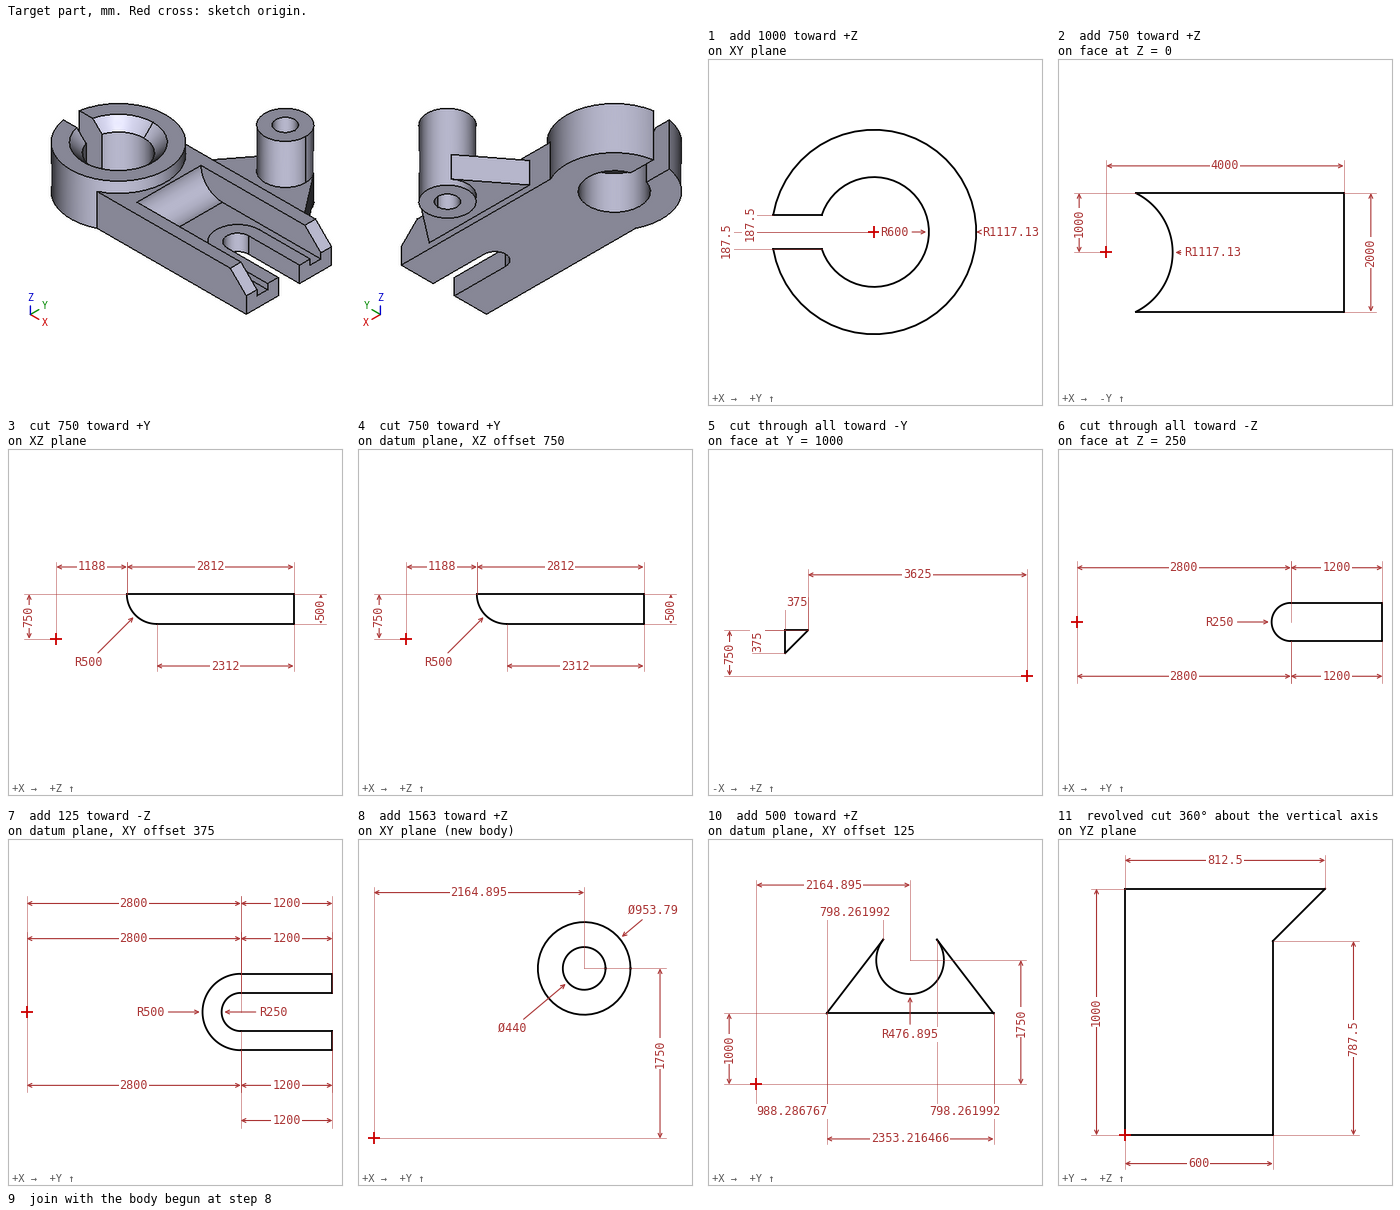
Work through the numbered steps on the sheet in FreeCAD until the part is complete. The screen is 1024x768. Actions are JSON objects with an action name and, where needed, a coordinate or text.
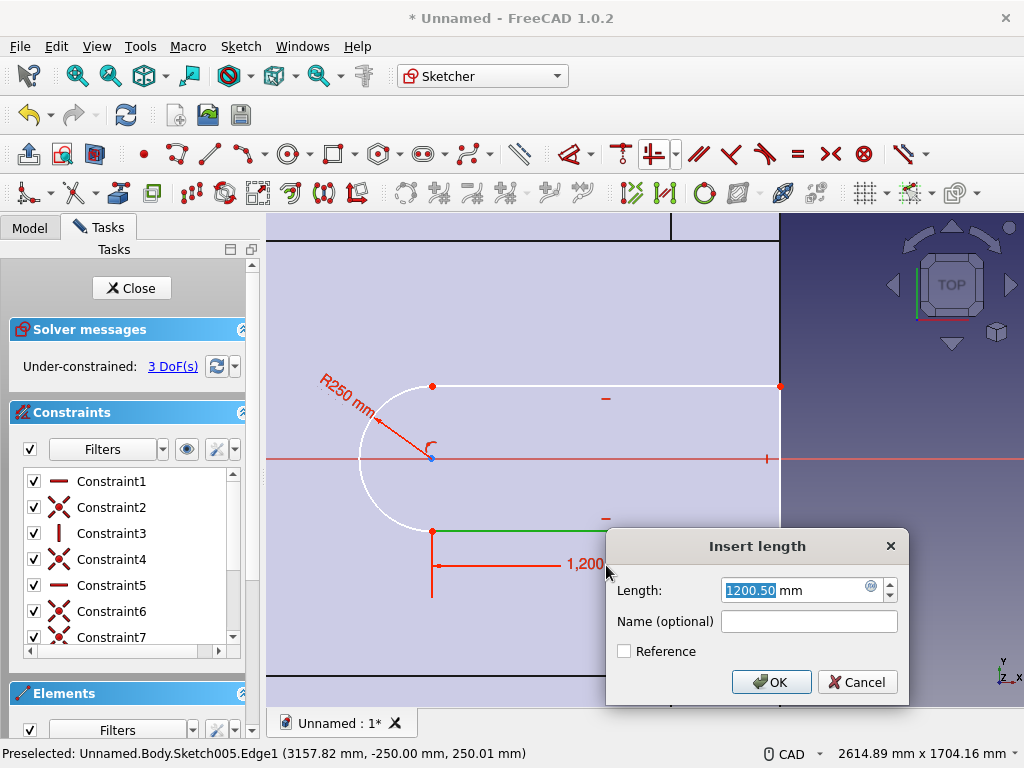
{"action": "type", "text": "1200"}
{"action": "key", "text": "Return"}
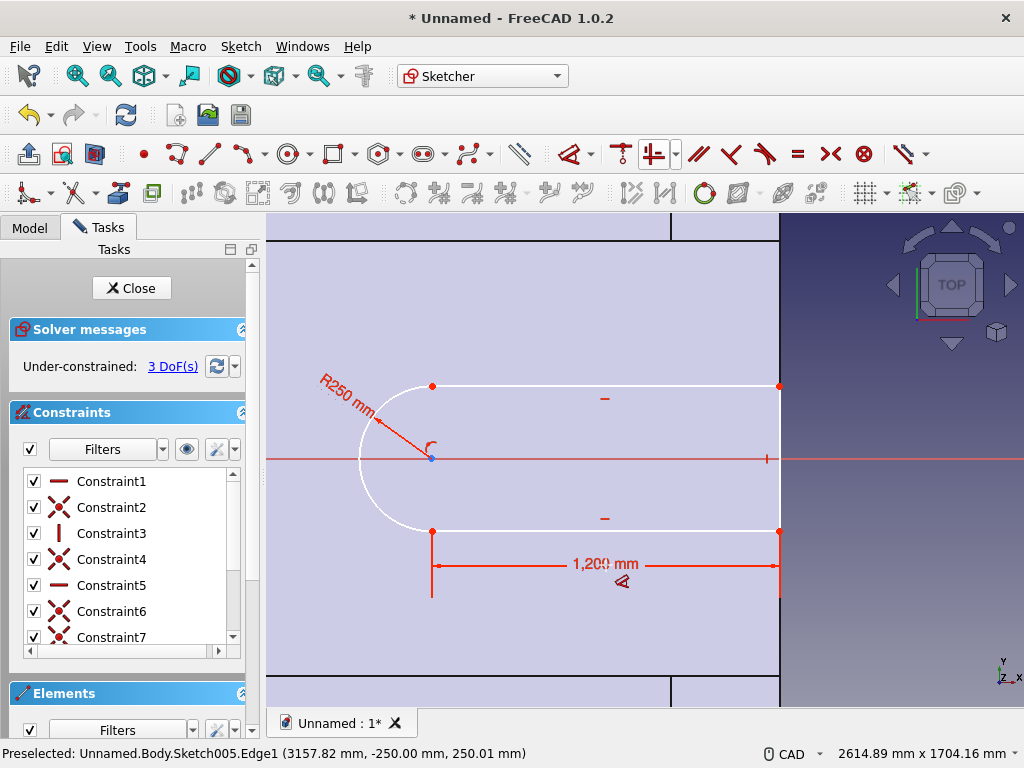
{"action": "left_click", "coordinate": [676, 386]}
{"action": "left_click", "coordinate": [606, 352]}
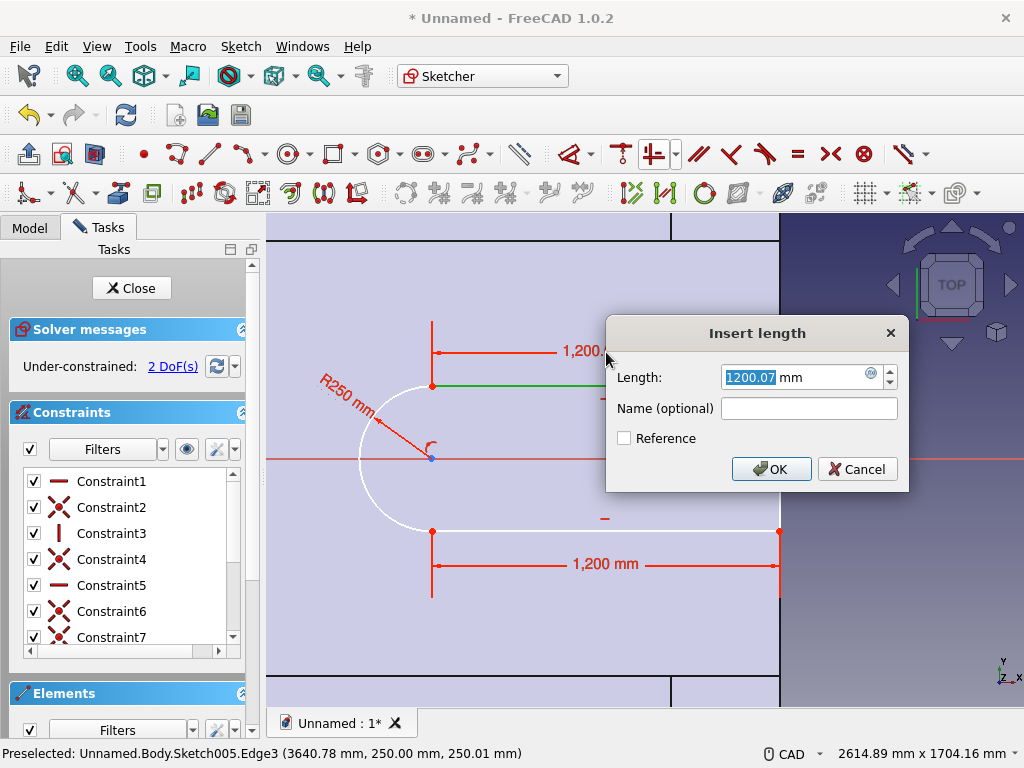
{"action": "type", "text": "1200"}
{"action": "key", "text": "Return"}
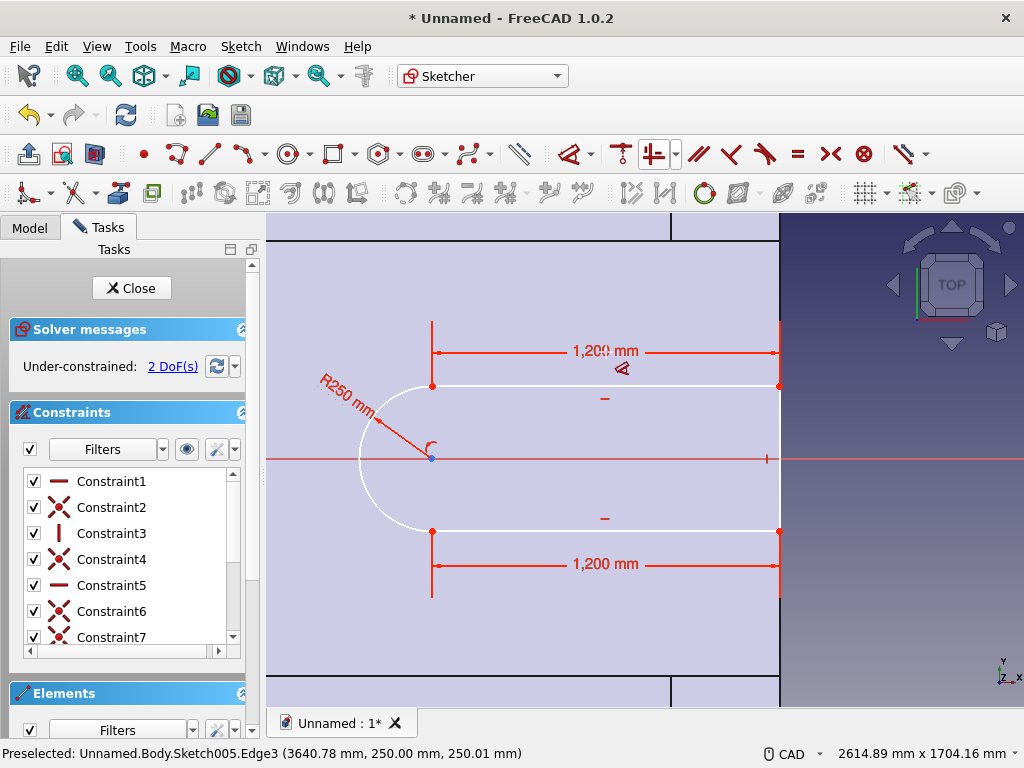
{"action": "left_click", "coordinate": [432, 531]}
{"action": "left_click", "coordinate": [363, 565]}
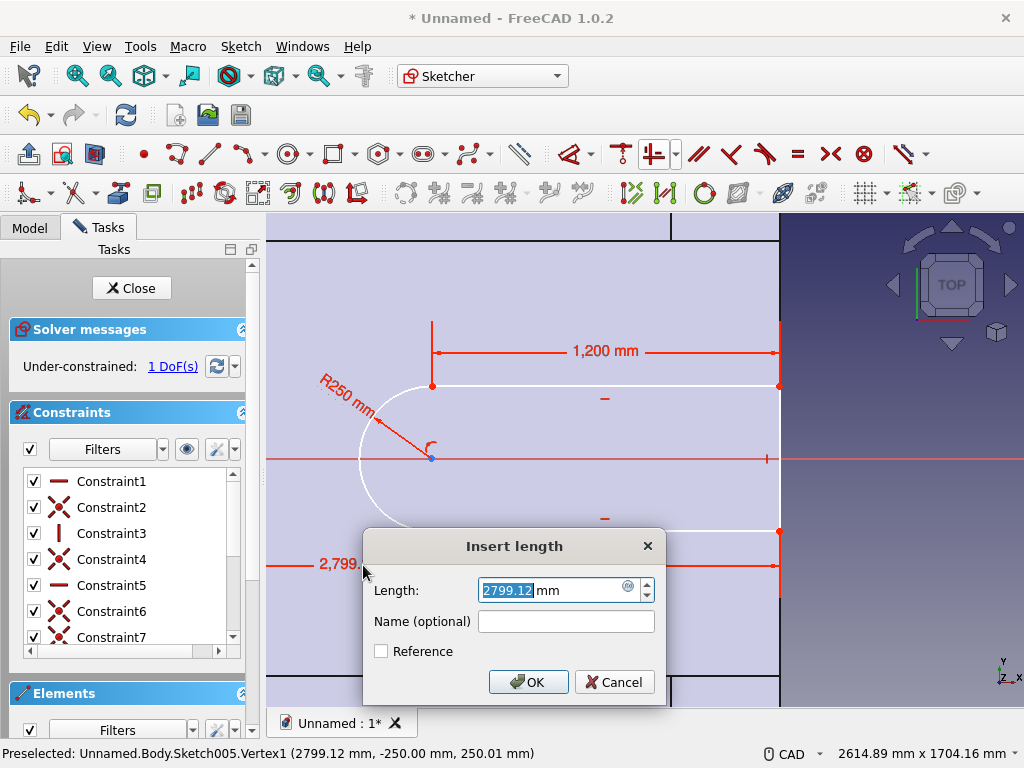
{"action": "type", "text": "2800"}
{"action": "key", "text": "Return"}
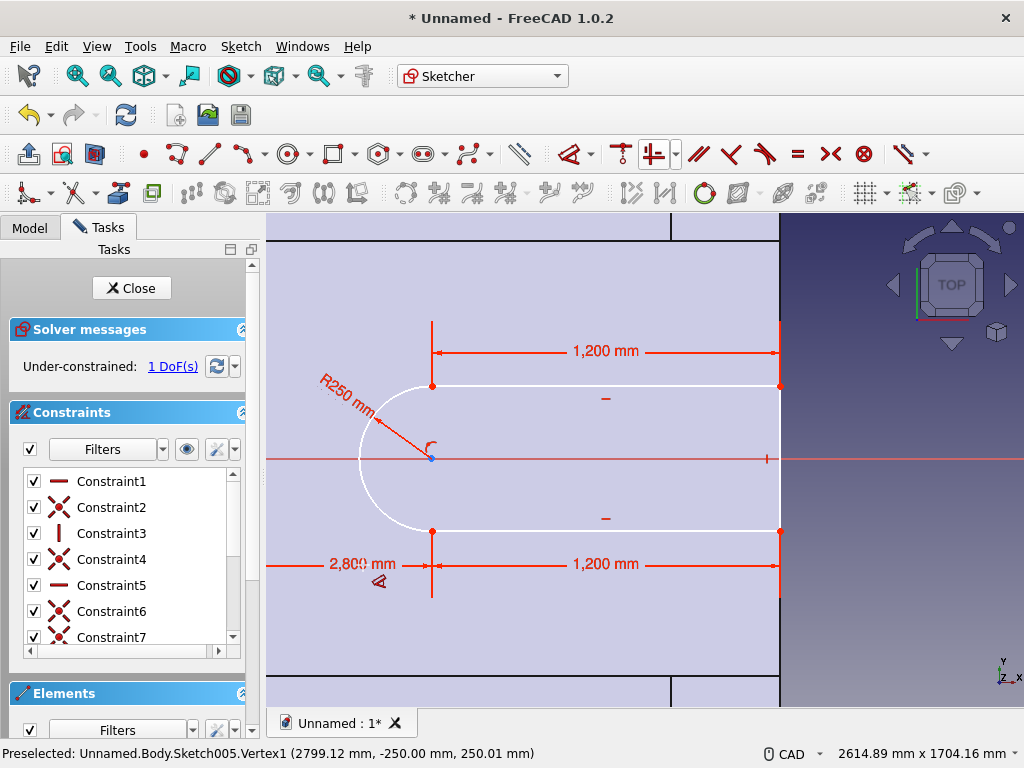
{"action": "left_click", "coordinate": [432, 459]}
{"action": "left_click", "coordinate": [331, 493]}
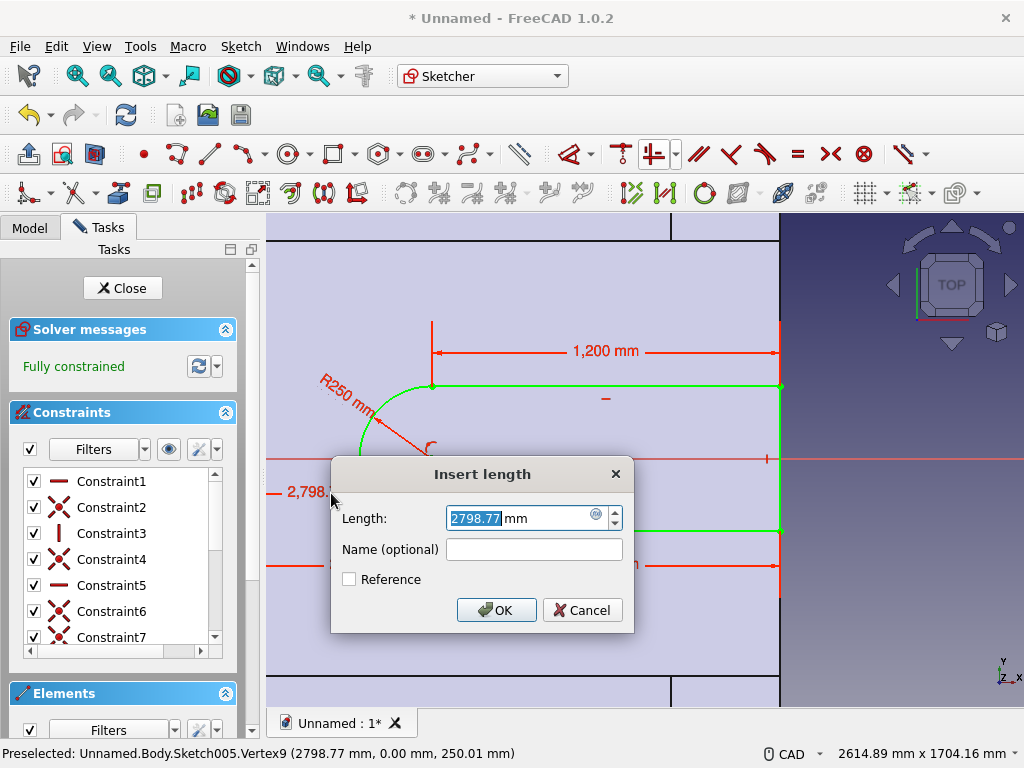
{"action": "type", "text": "2800"}
{"action": "key", "text": "Return"}
{"action": "key", "text": "Escape"}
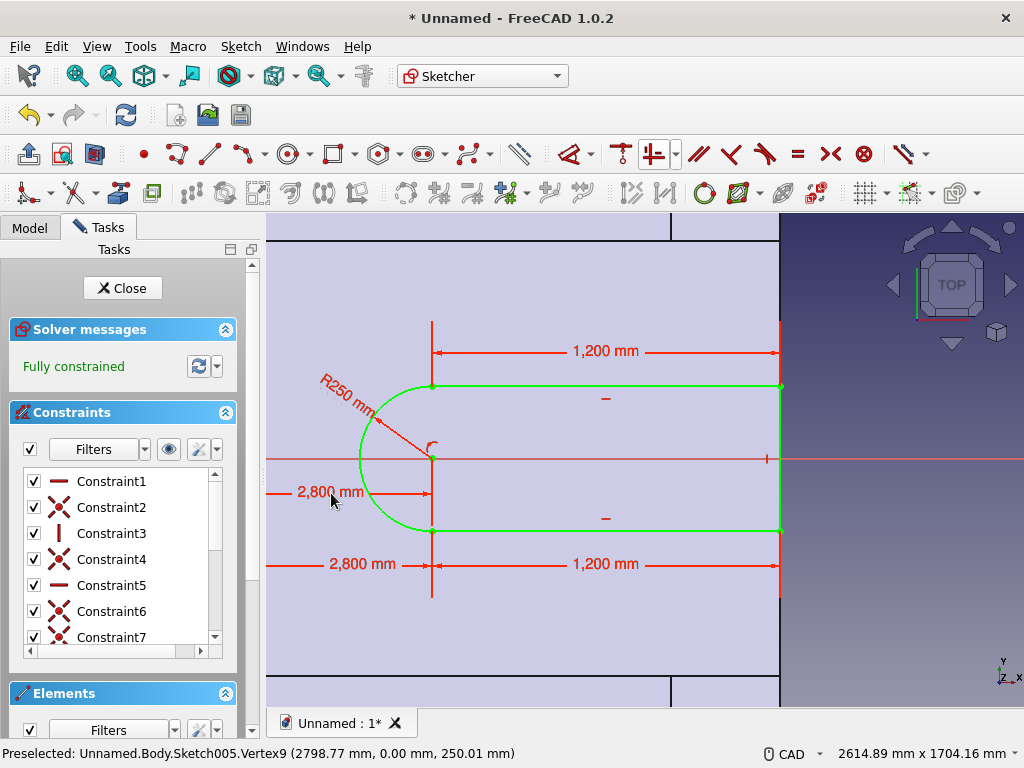
{"action": "left_click", "coordinate": [123, 288]}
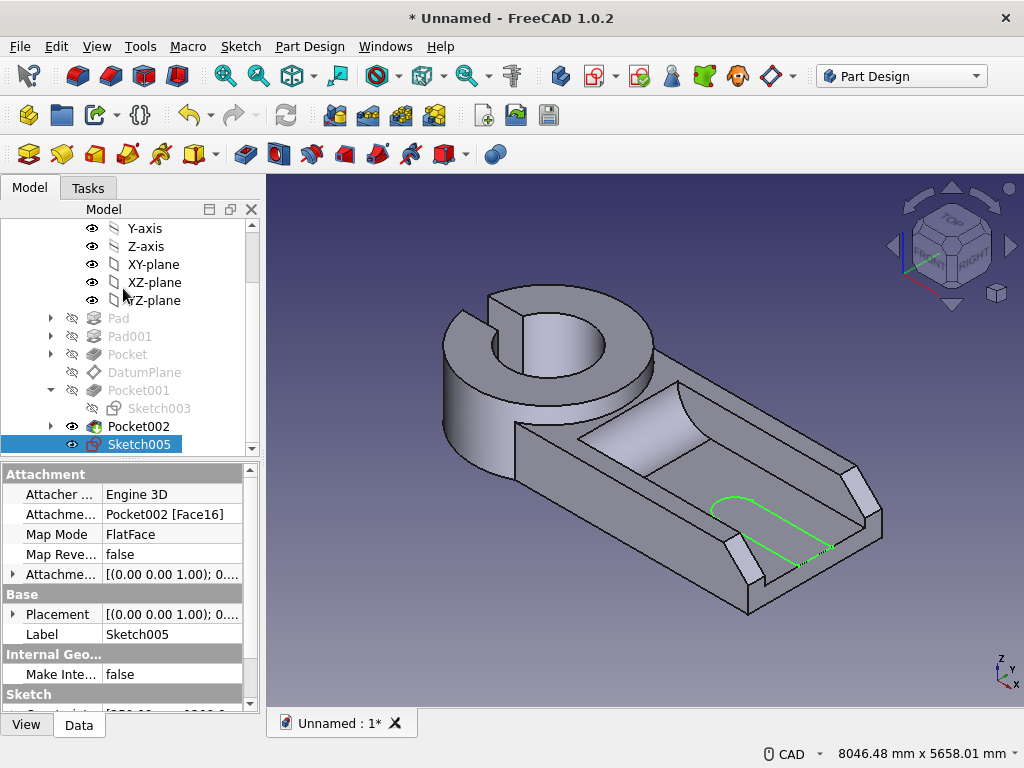
{"action": "left_click", "coordinate": [246, 154]}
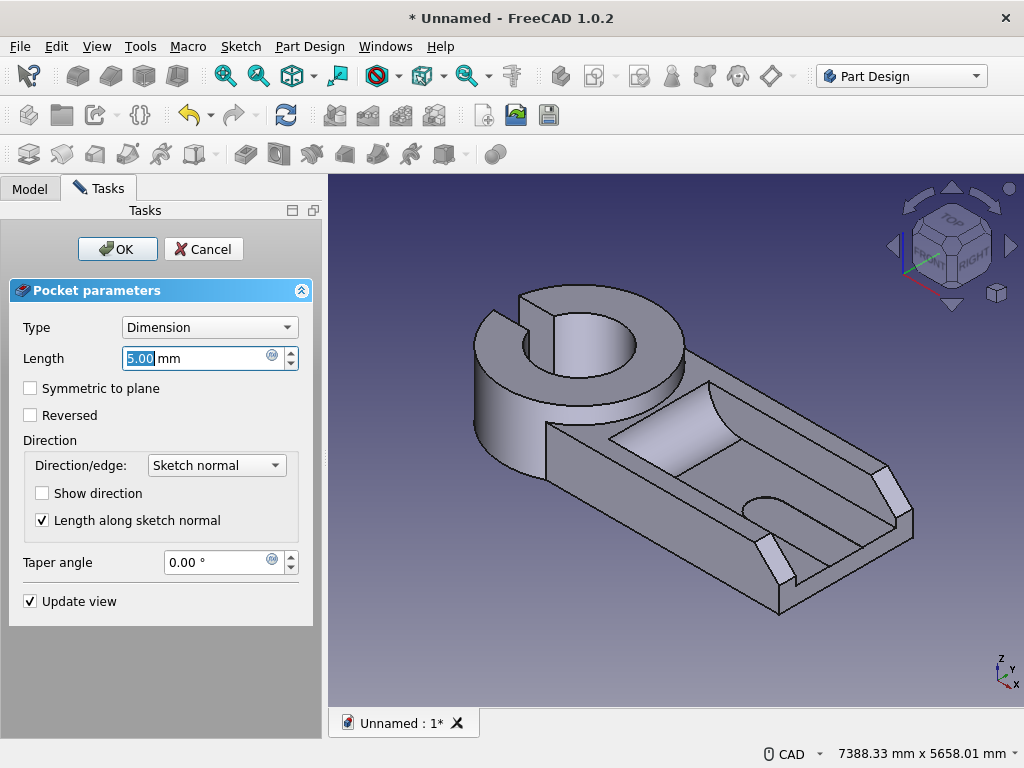
{"action": "left_click", "coordinate": [210, 328]}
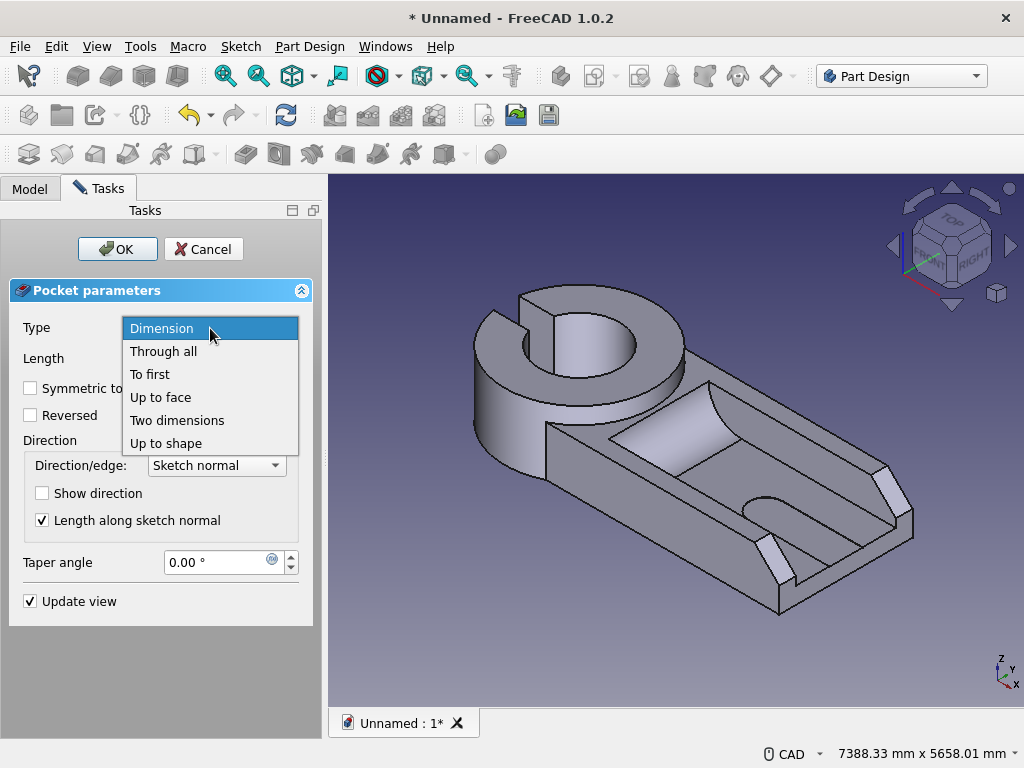
{"action": "left_click", "coordinate": [208, 352]}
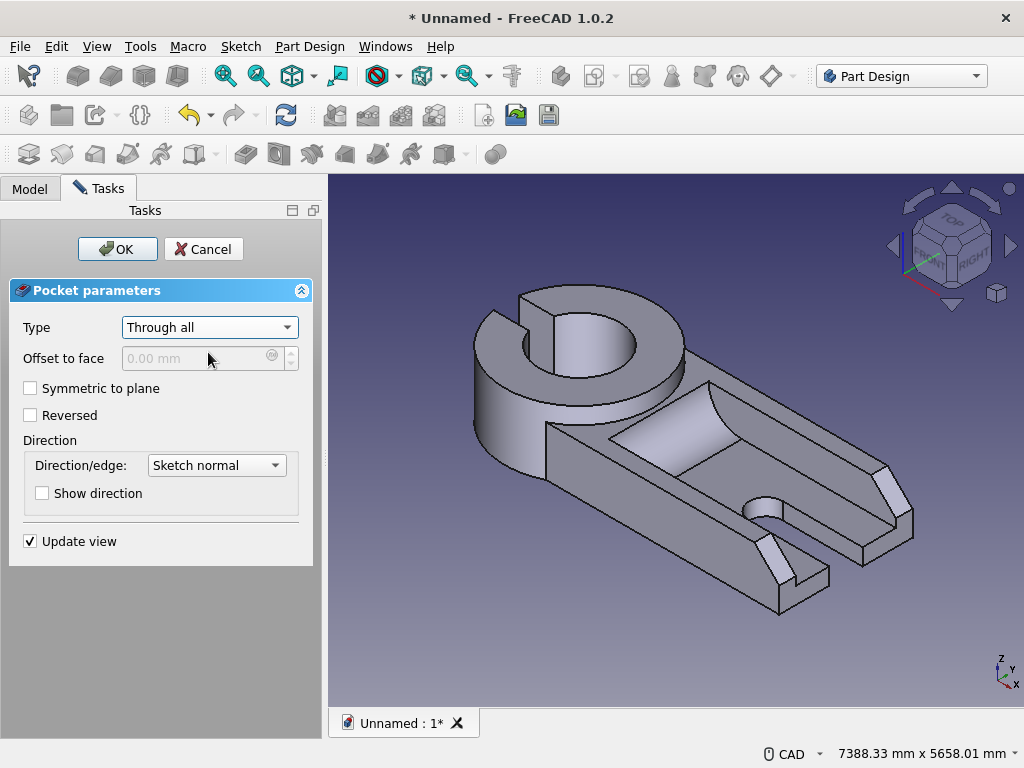
{"action": "left_click", "coordinate": [118, 249]}